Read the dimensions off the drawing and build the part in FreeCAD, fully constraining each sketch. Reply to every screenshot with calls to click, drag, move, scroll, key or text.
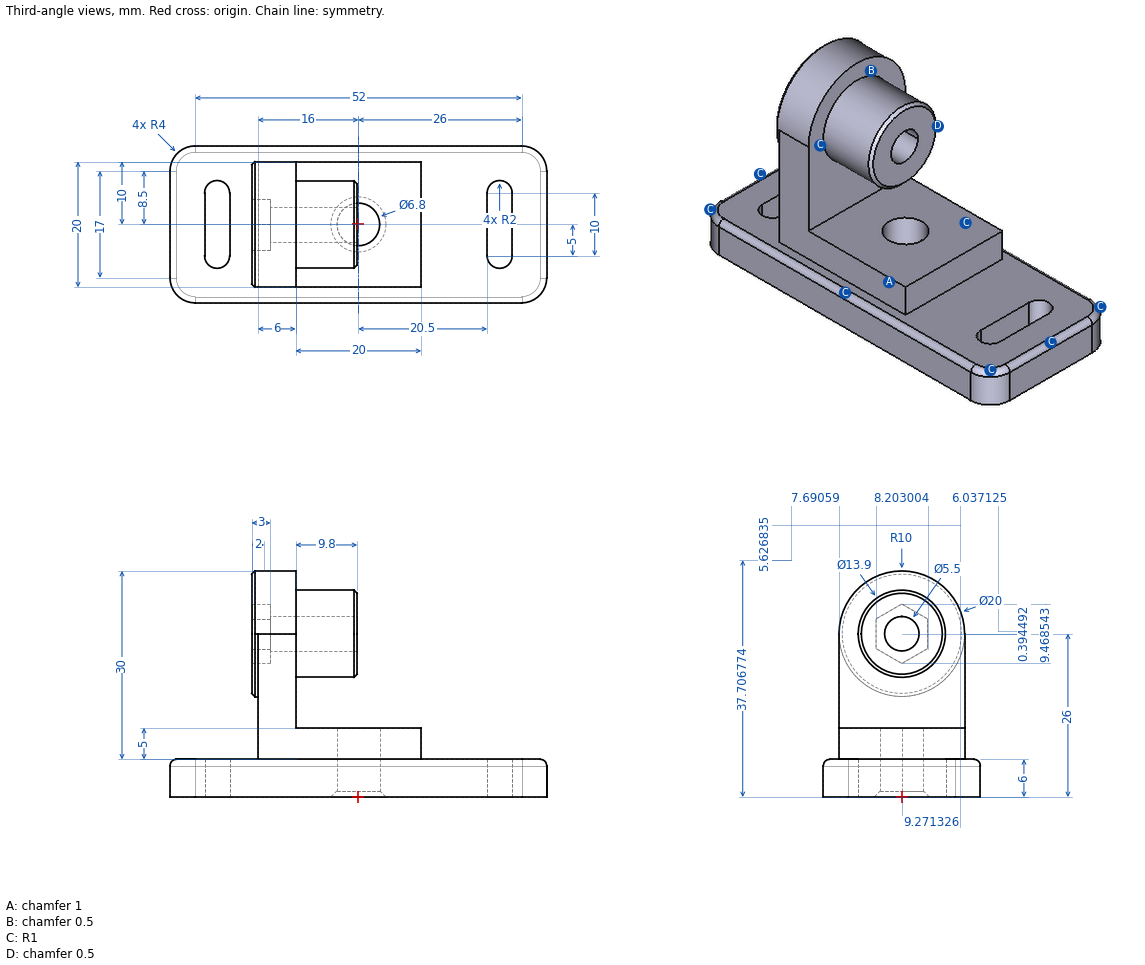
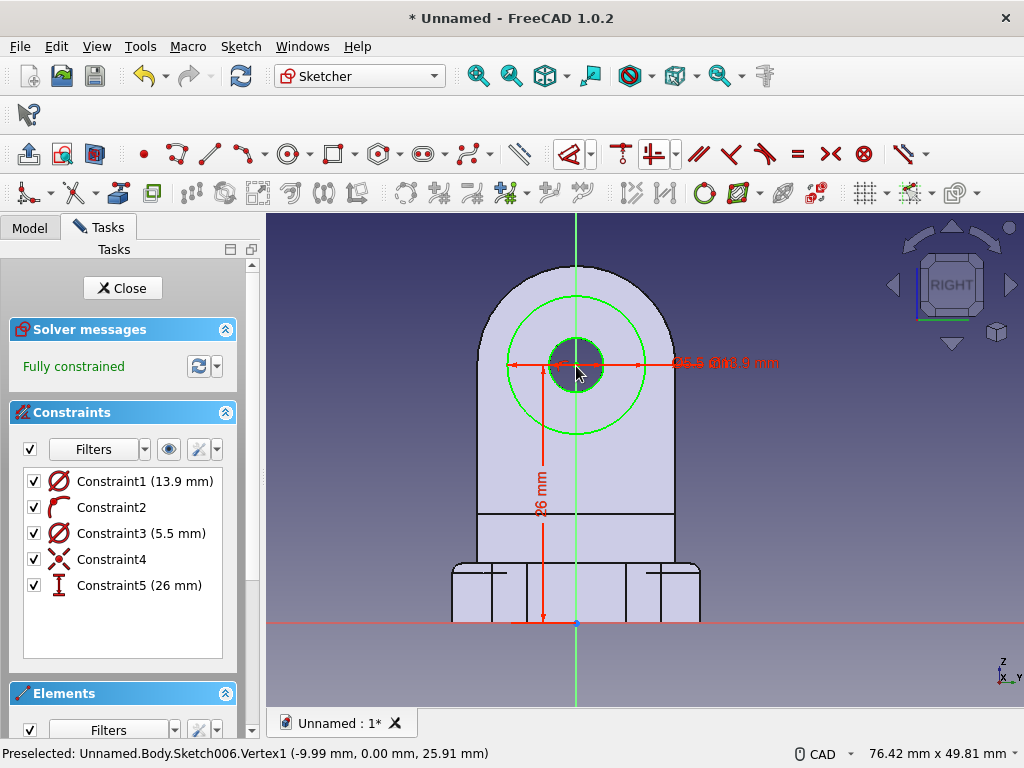
click(123, 288)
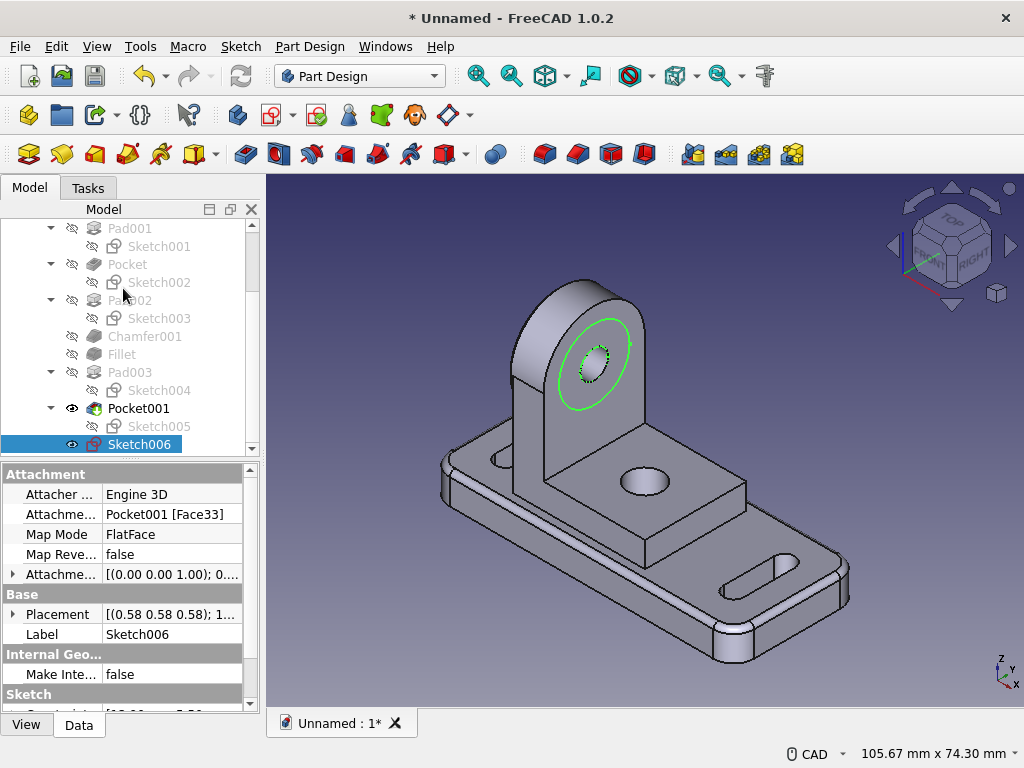
click(29, 154)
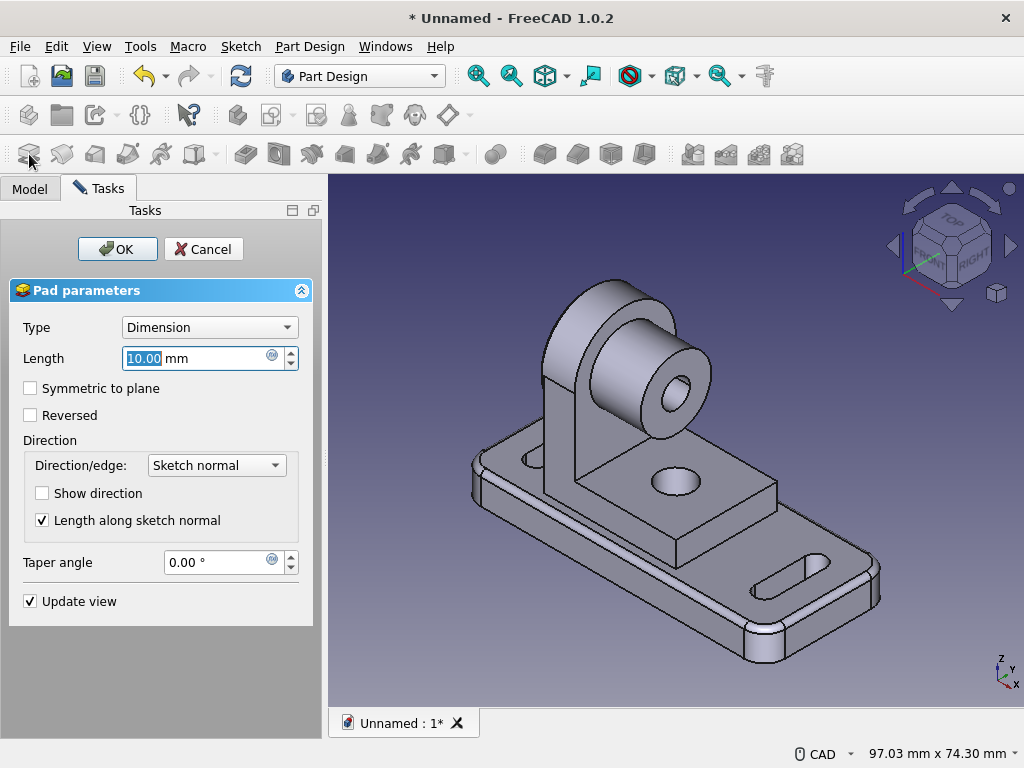
text(9.8)
key(Tab)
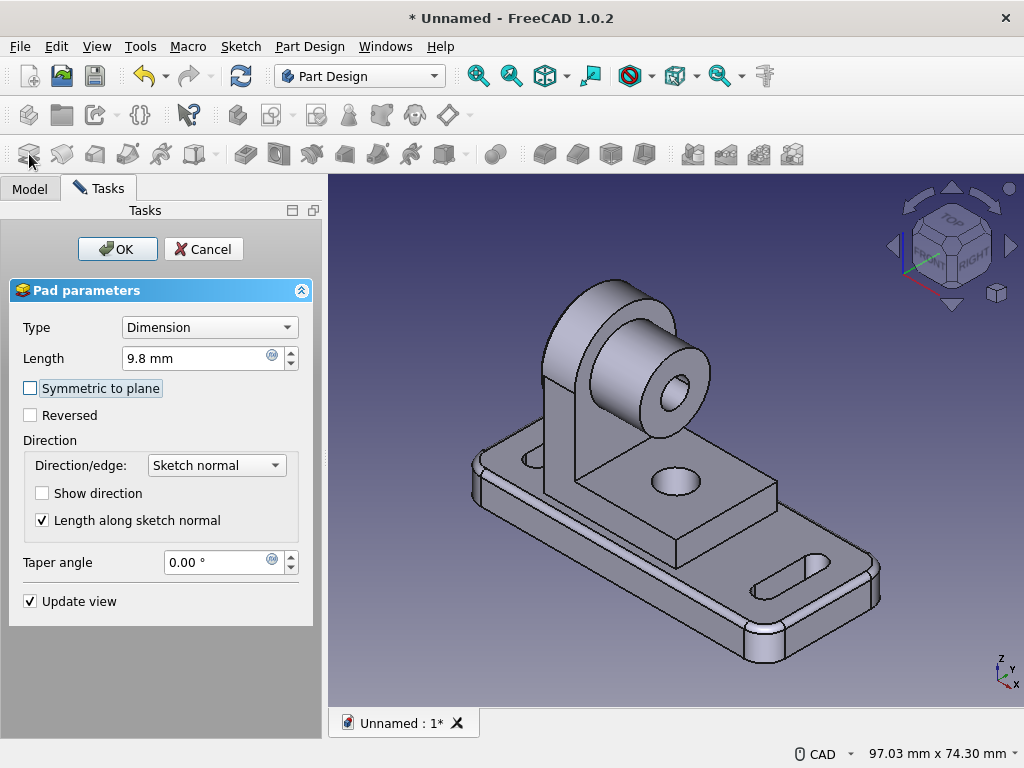
click(118, 249)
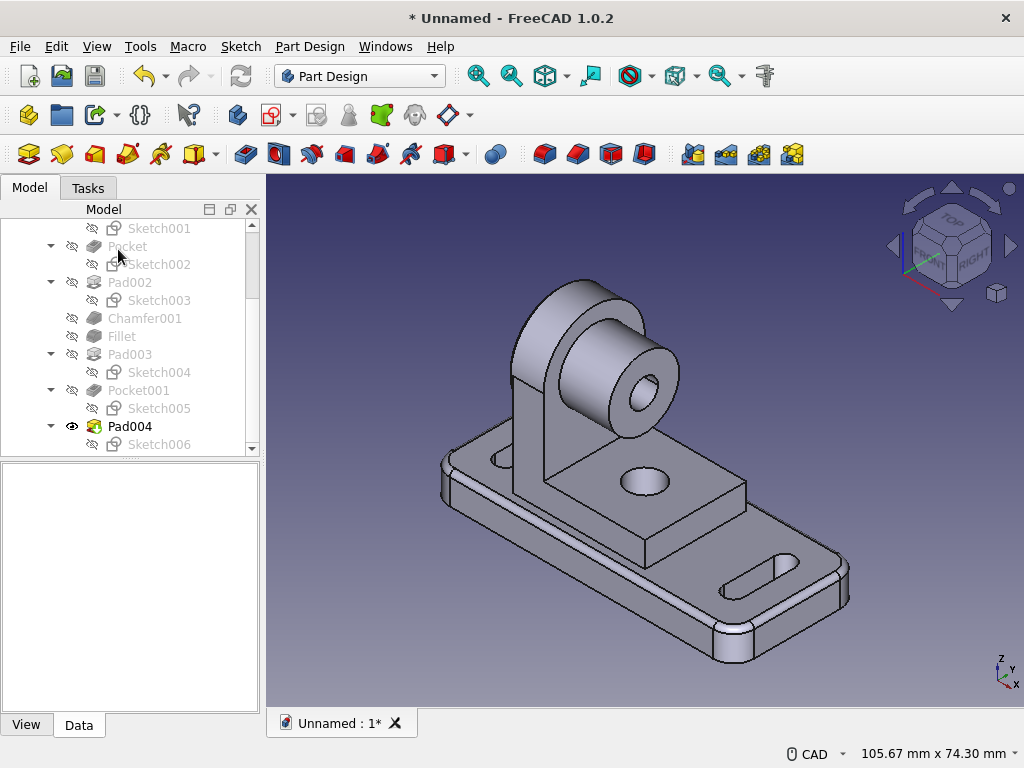
click(609, 412)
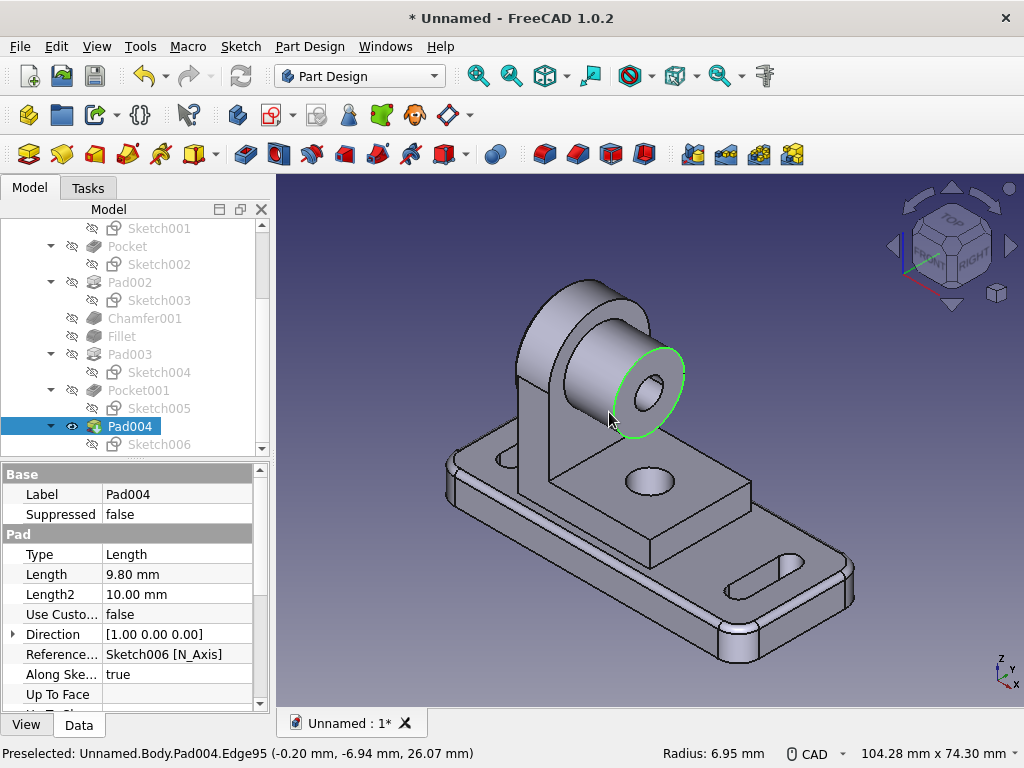
click(578, 154)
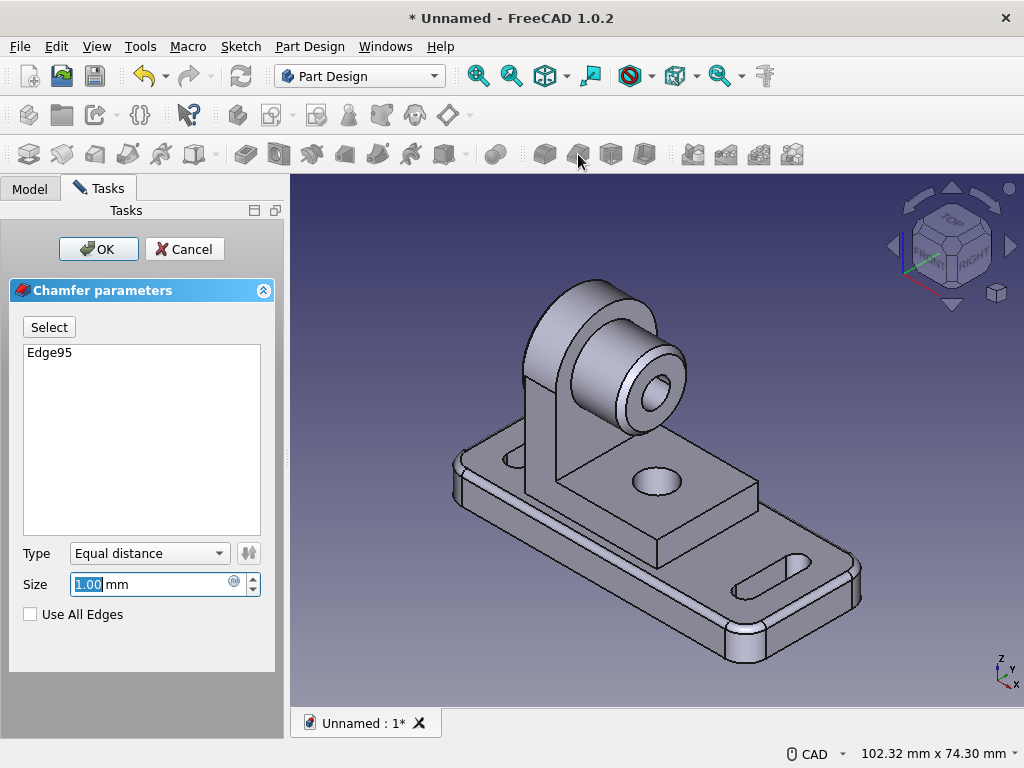
text(0.5)
key(Tab)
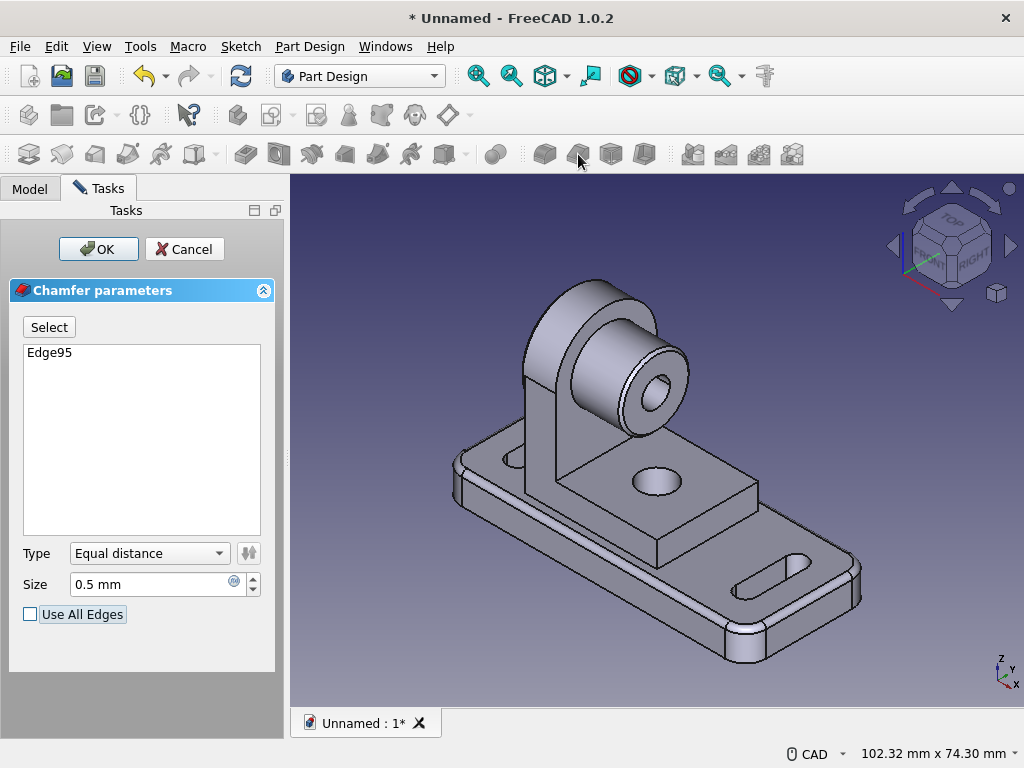
click(99, 249)